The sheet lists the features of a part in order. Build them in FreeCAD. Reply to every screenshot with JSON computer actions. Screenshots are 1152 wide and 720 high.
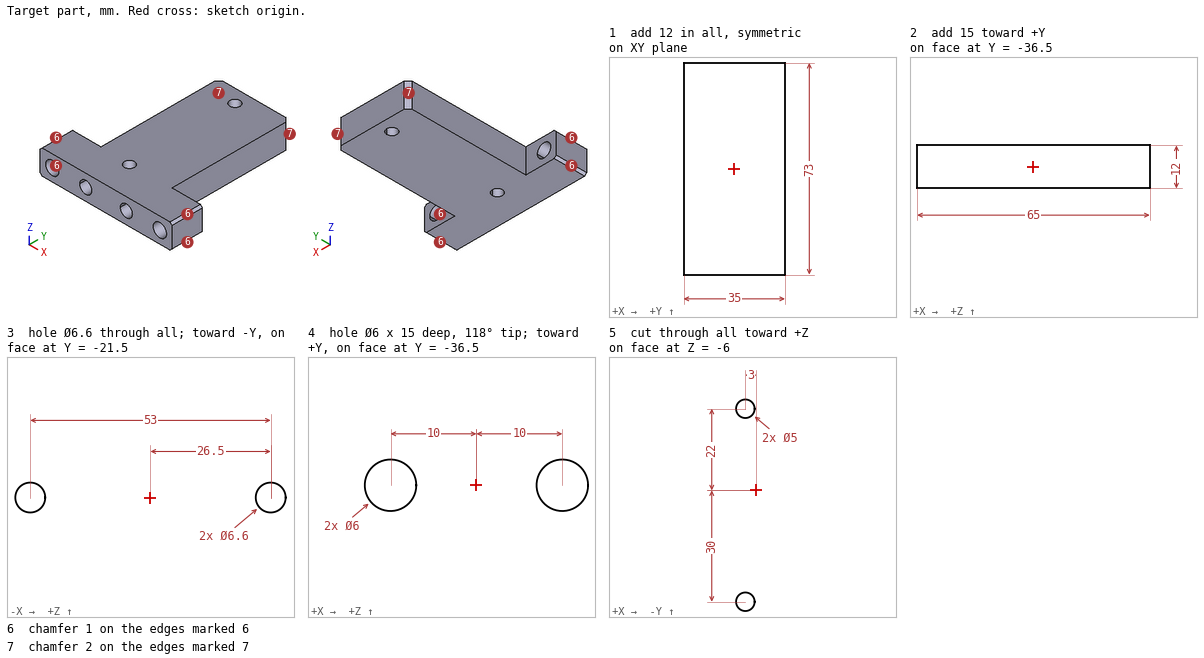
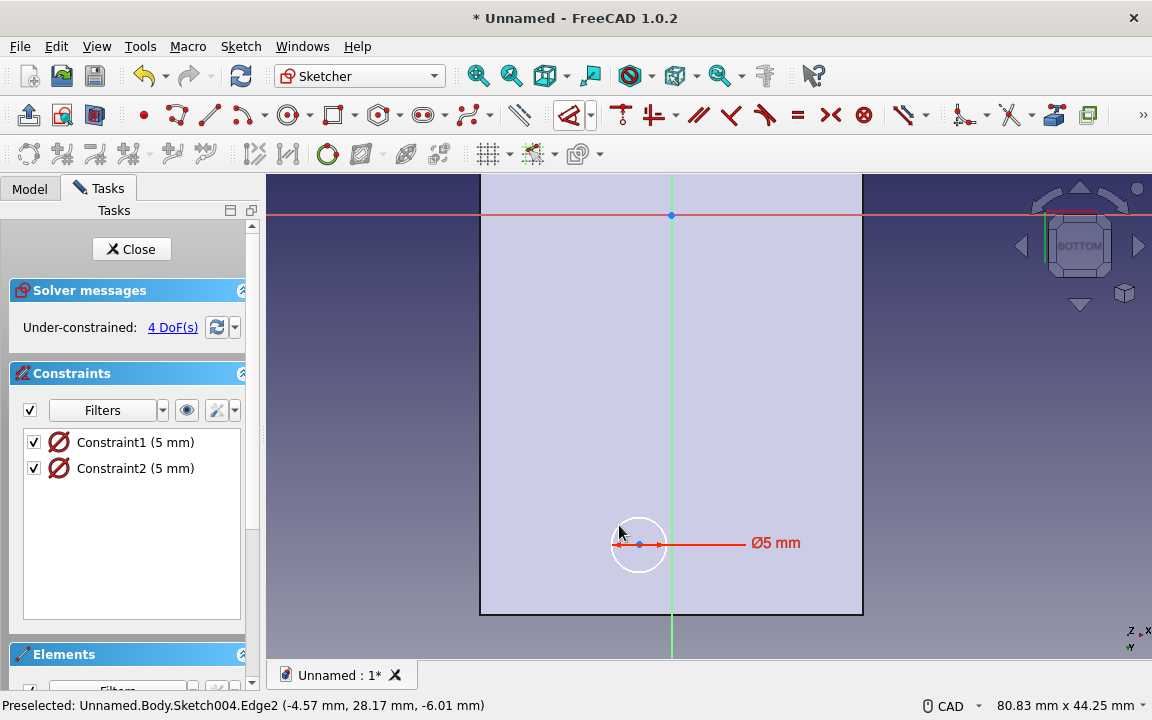
{"action": "scroll", "coordinate": [640, 545], "scroll_direction": "down", "scroll_amount": 4}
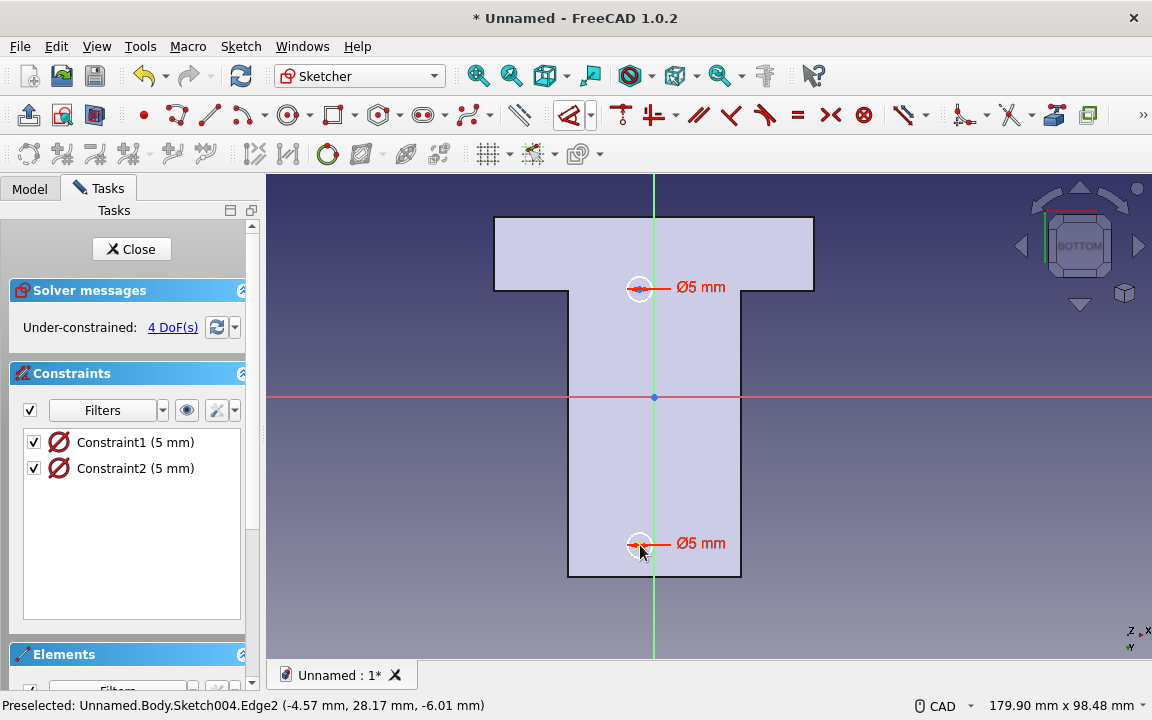
{"action": "left_click", "coordinate": [640, 289]}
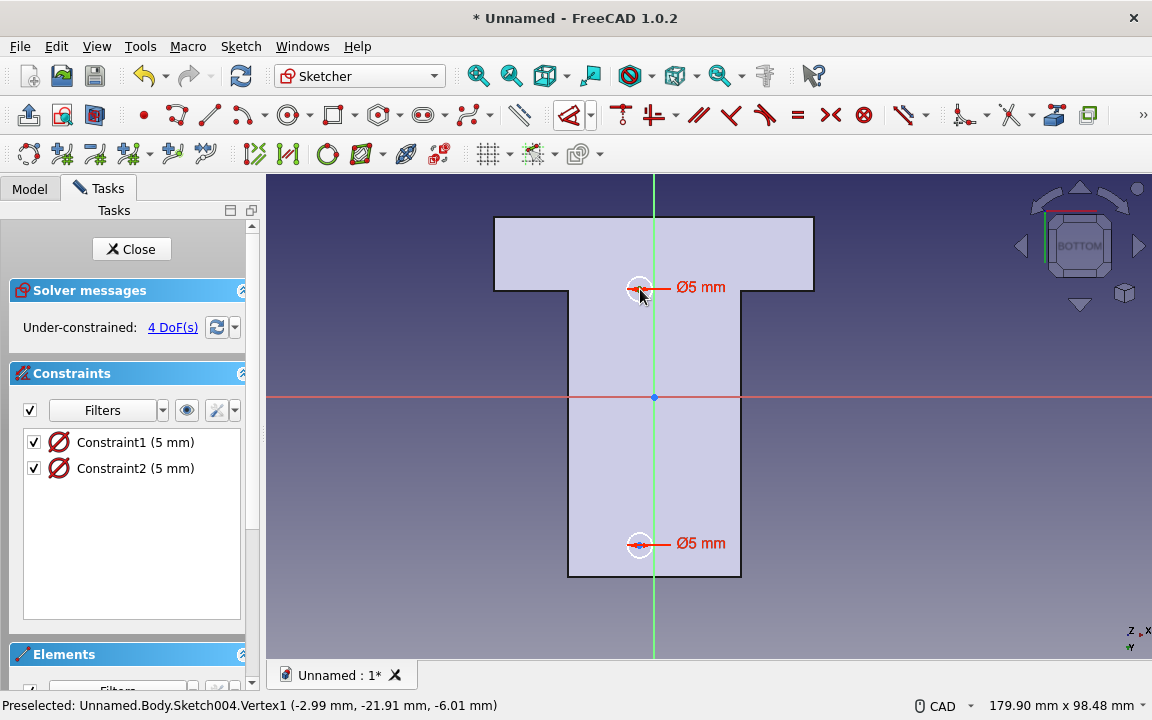
{"action": "left_click", "coordinate": [640, 545]}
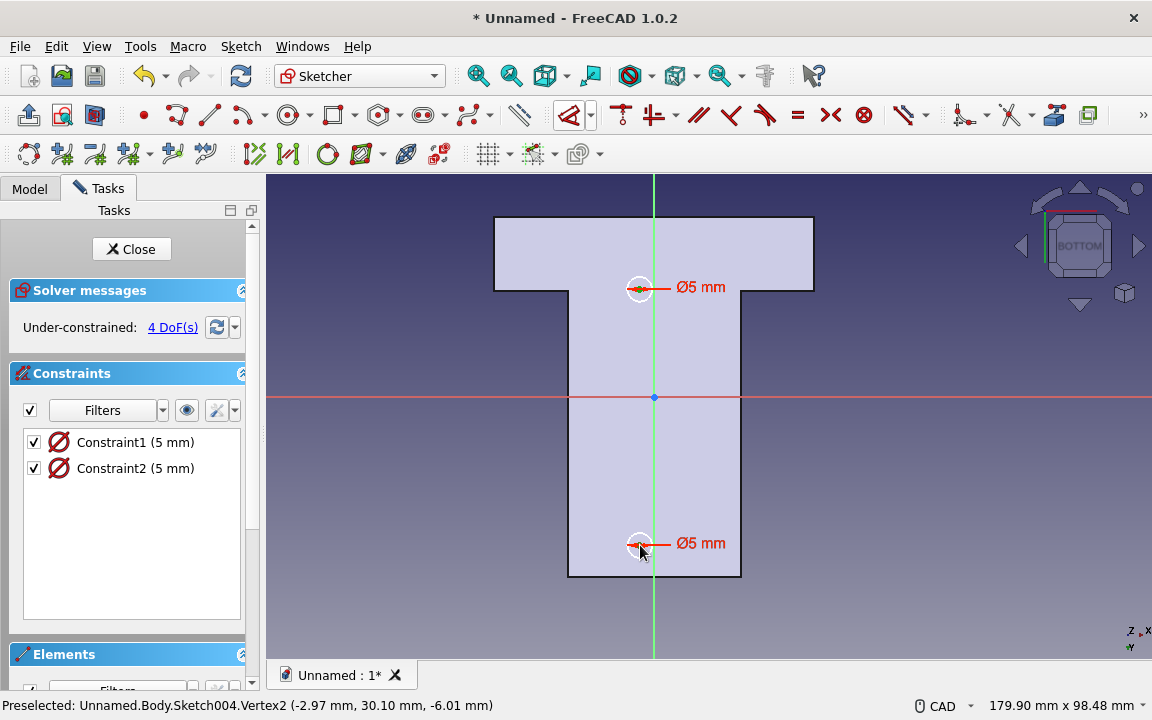
{"action": "key", "text": "v"}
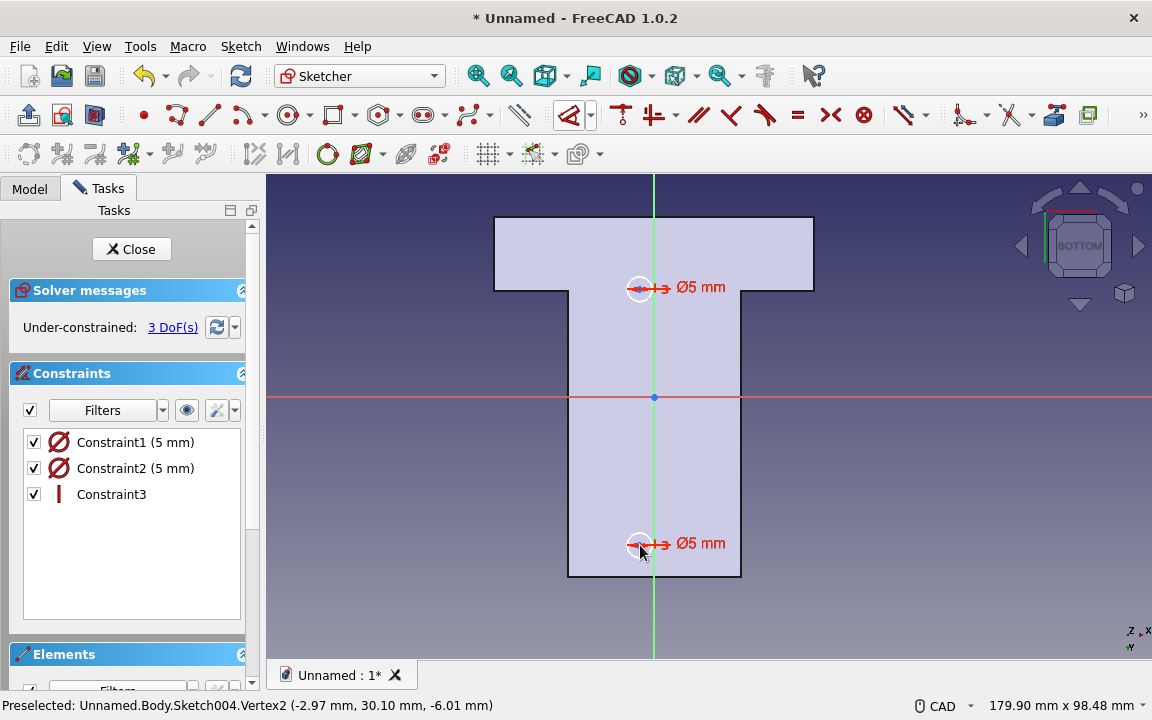
{"action": "scroll", "coordinate": [640, 289], "scroll_direction": "up", "scroll_amount": 5}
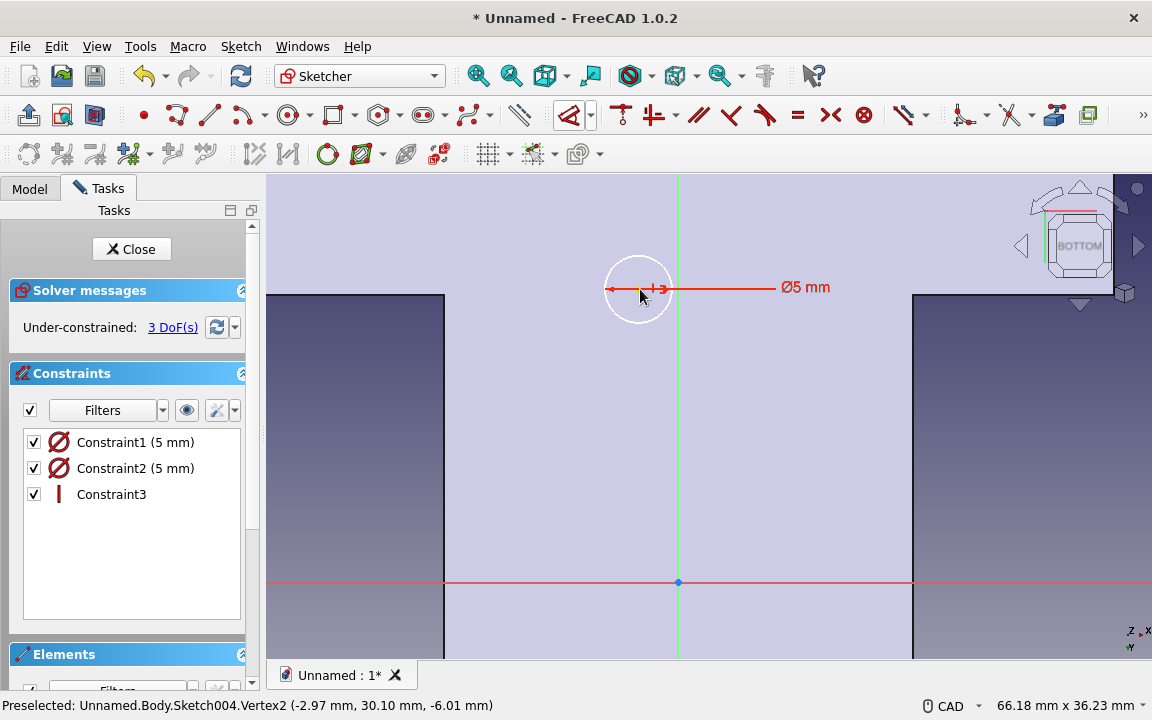
{"action": "left_click", "coordinate": [638, 289]}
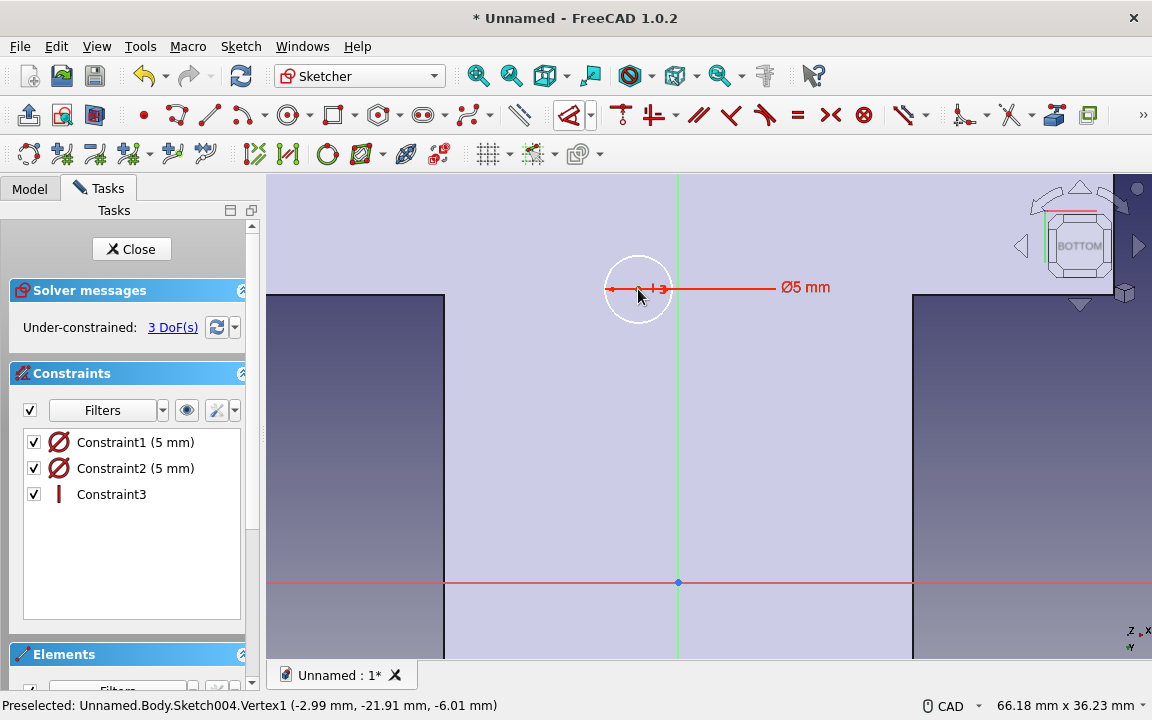
{"action": "left_click", "coordinate": [590, 116]}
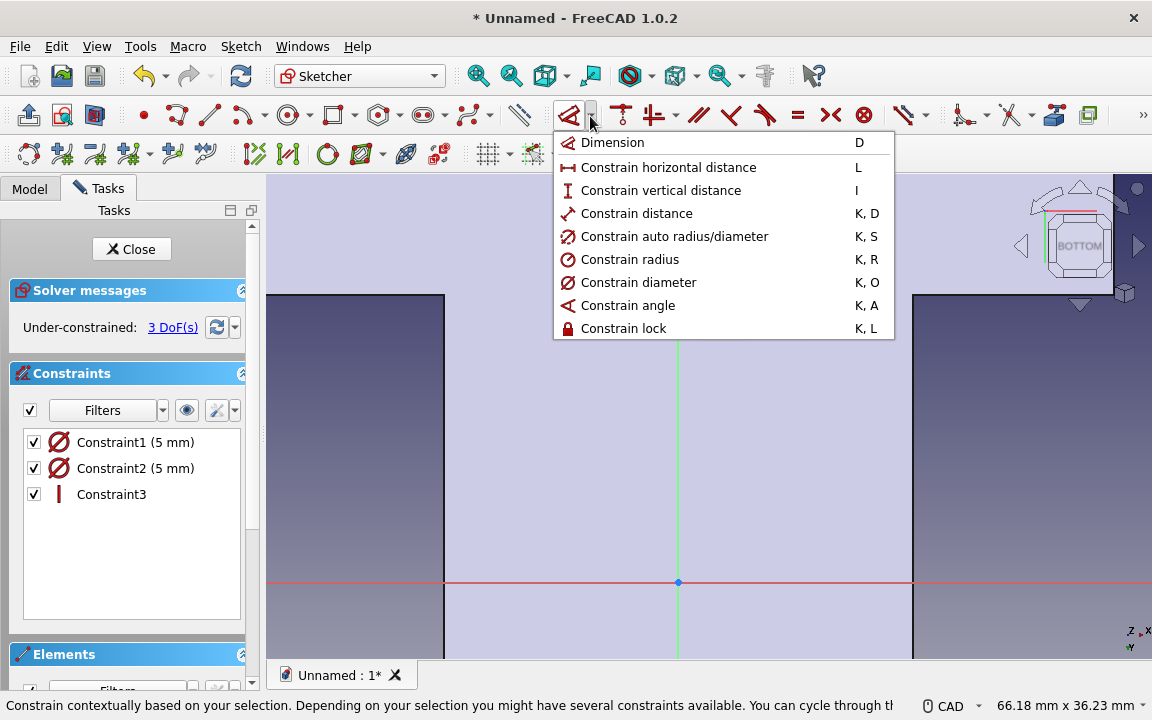
{"action": "left_click", "coordinate": [724, 168]}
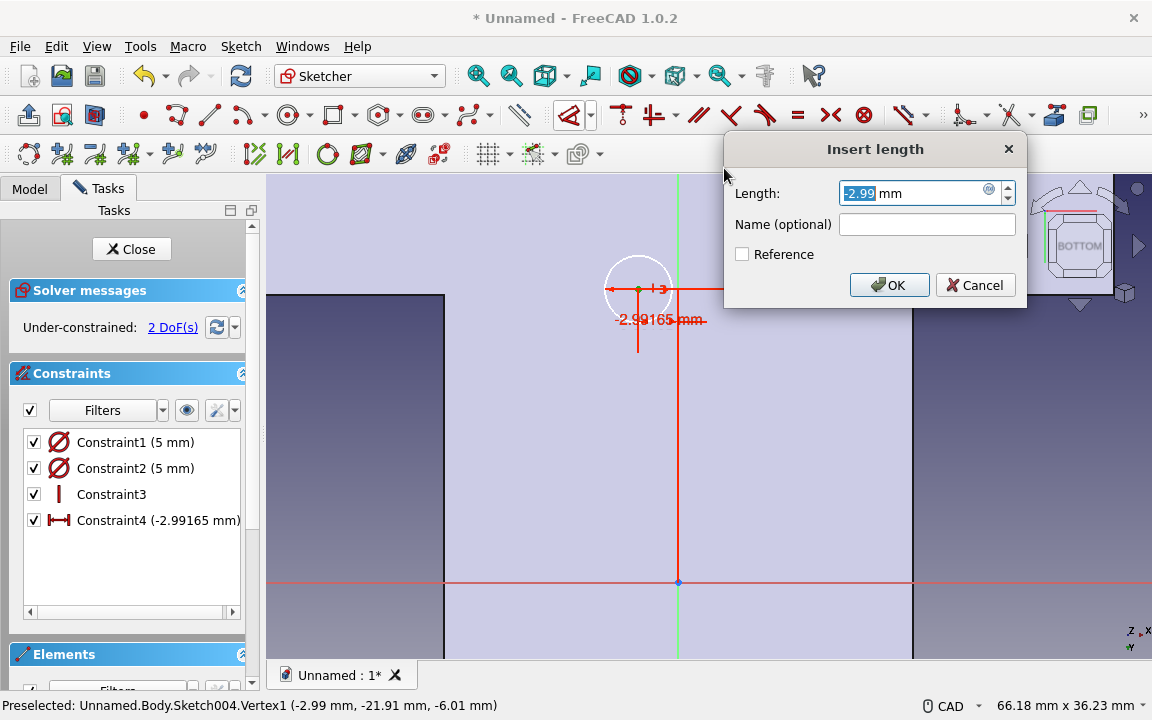
{"action": "type", "text": "-3"}
{"action": "key", "text": "Return"}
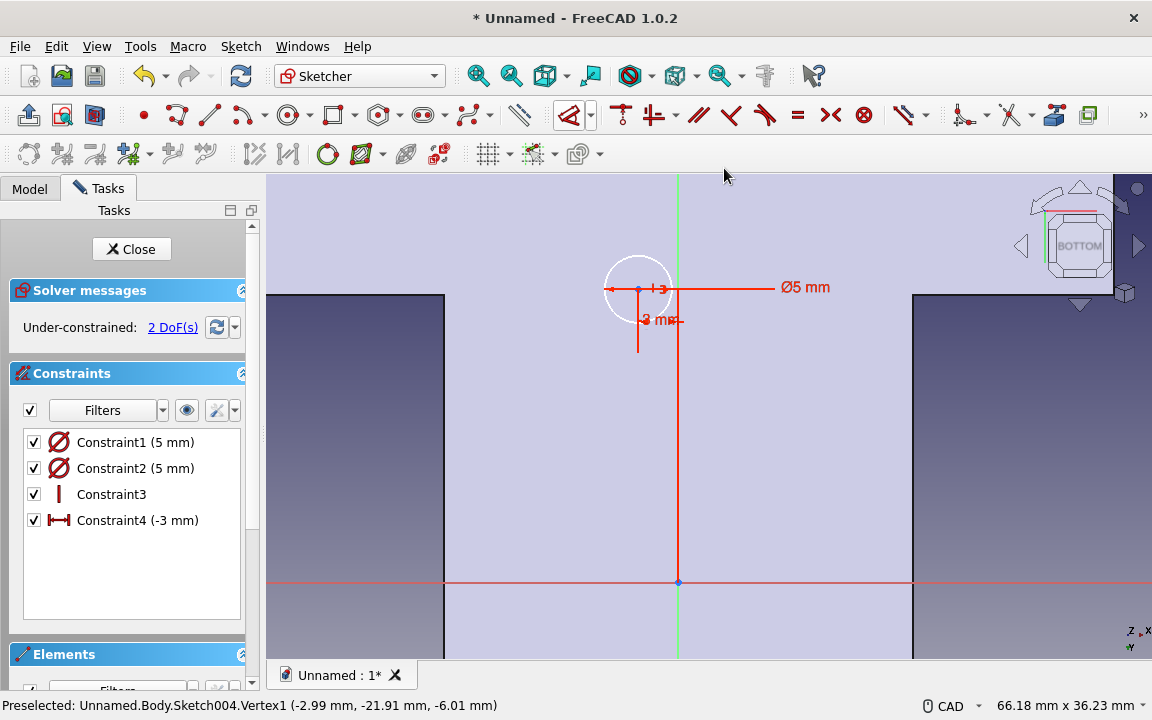
{"action": "left_click", "coordinate": [638, 289]}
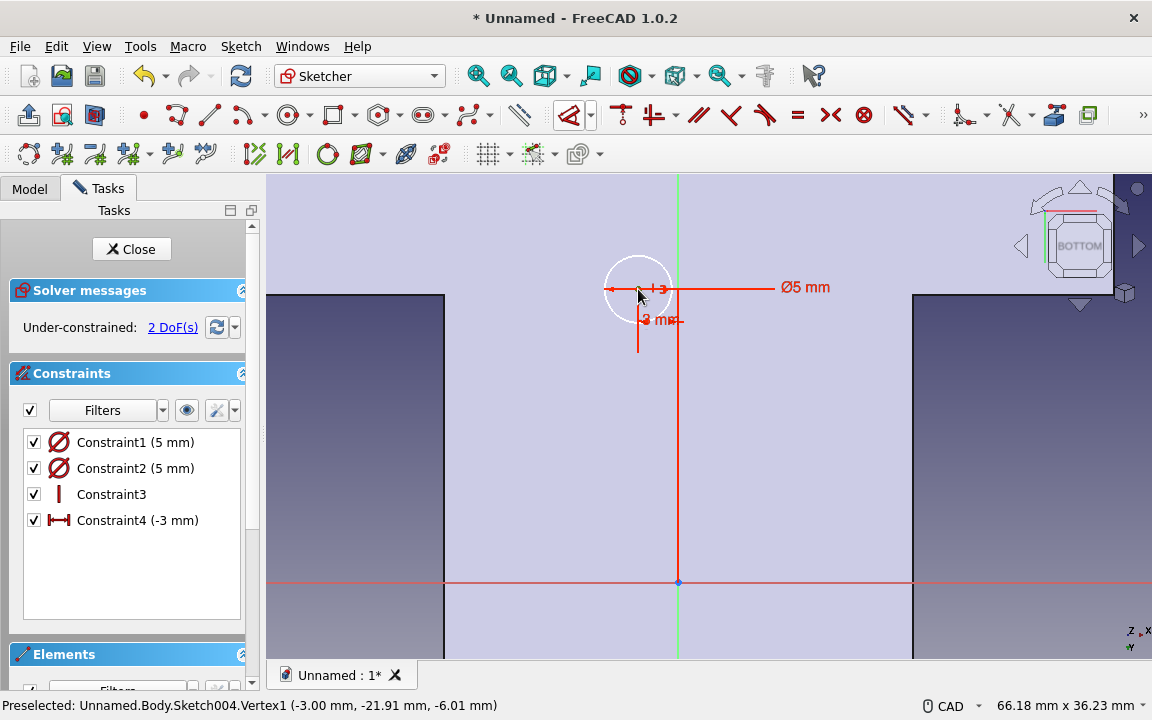
{"action": "key", "text": "i"}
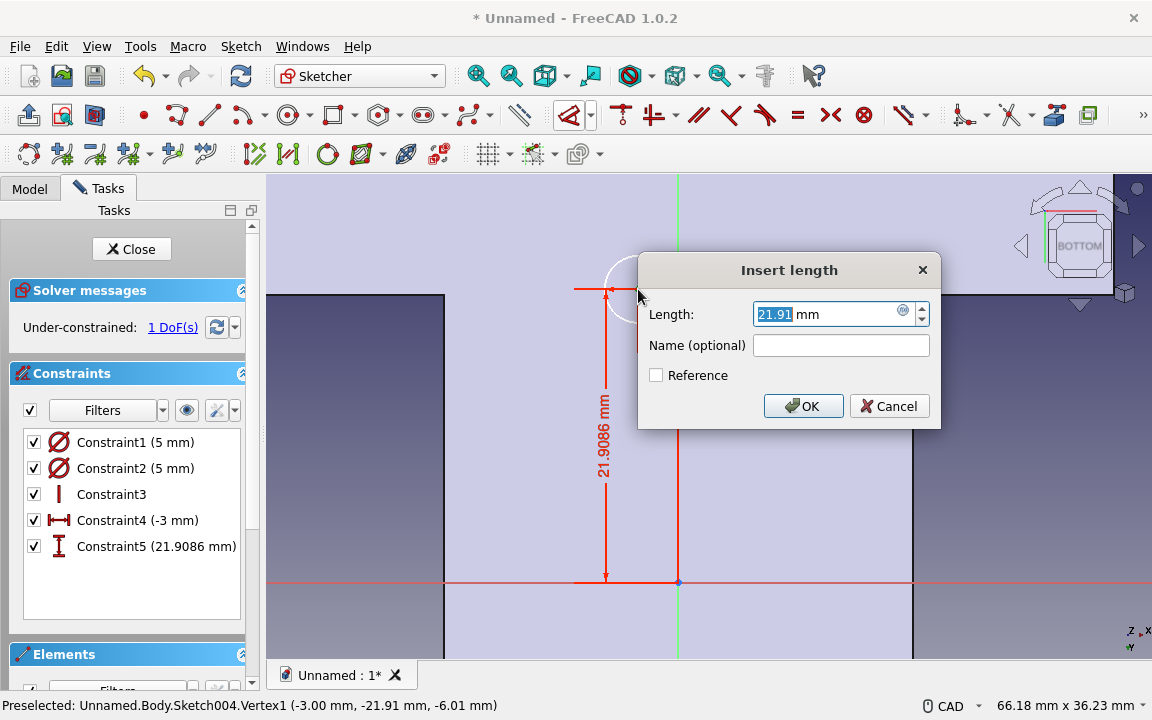
{"action": "type", "text": "22"}
{"action": "key", "text": "Return"}